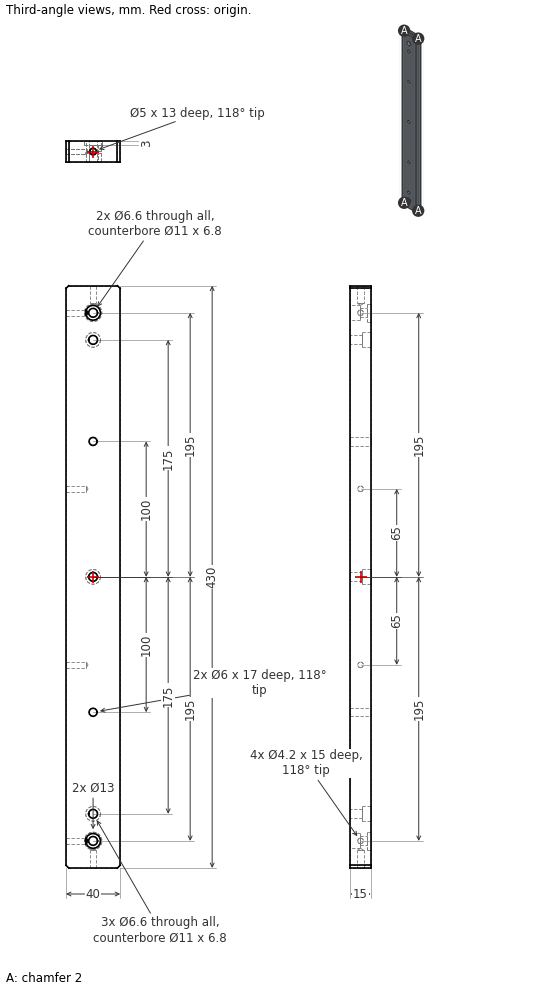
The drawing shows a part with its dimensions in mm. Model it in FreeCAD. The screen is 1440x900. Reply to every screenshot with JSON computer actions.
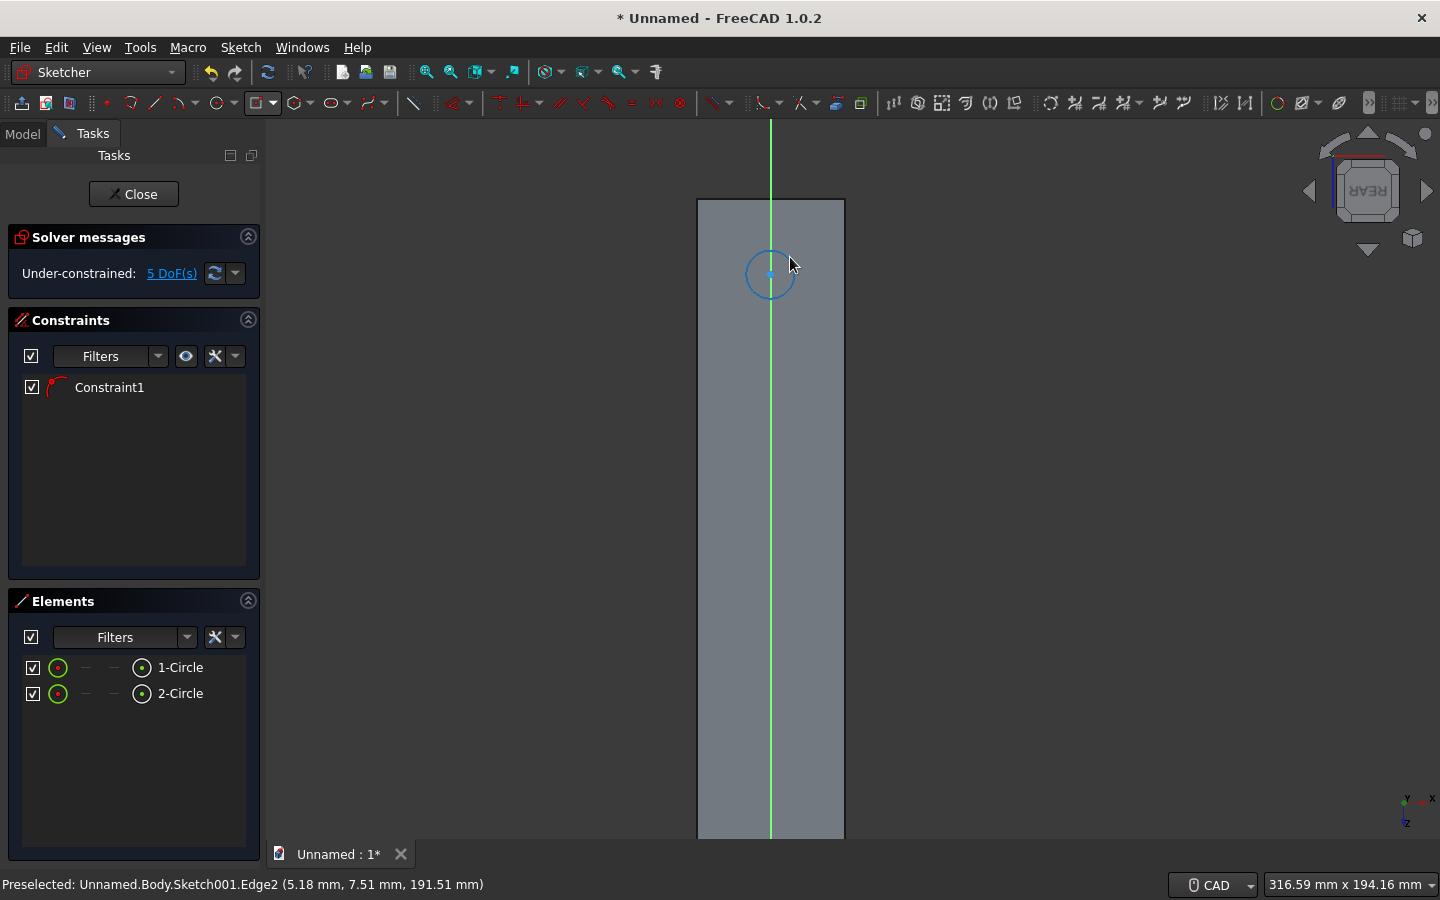
{"action": "left_click", "coordinate": [787, 258]}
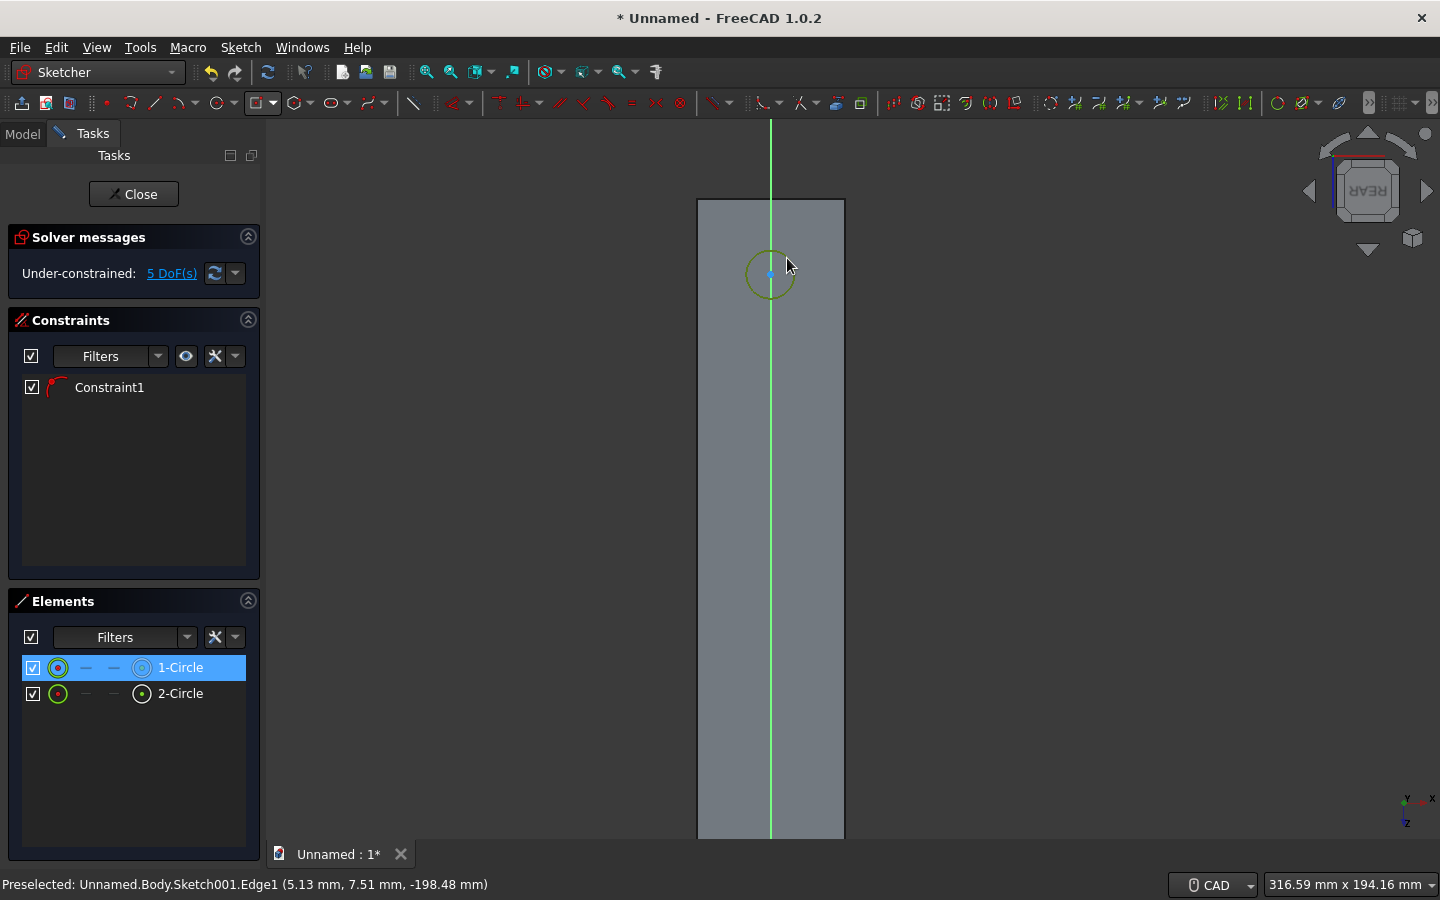
{"action": "scroll", "coordinate": [790, 256], "scroll_direction": "down", "scroll_amount": 6}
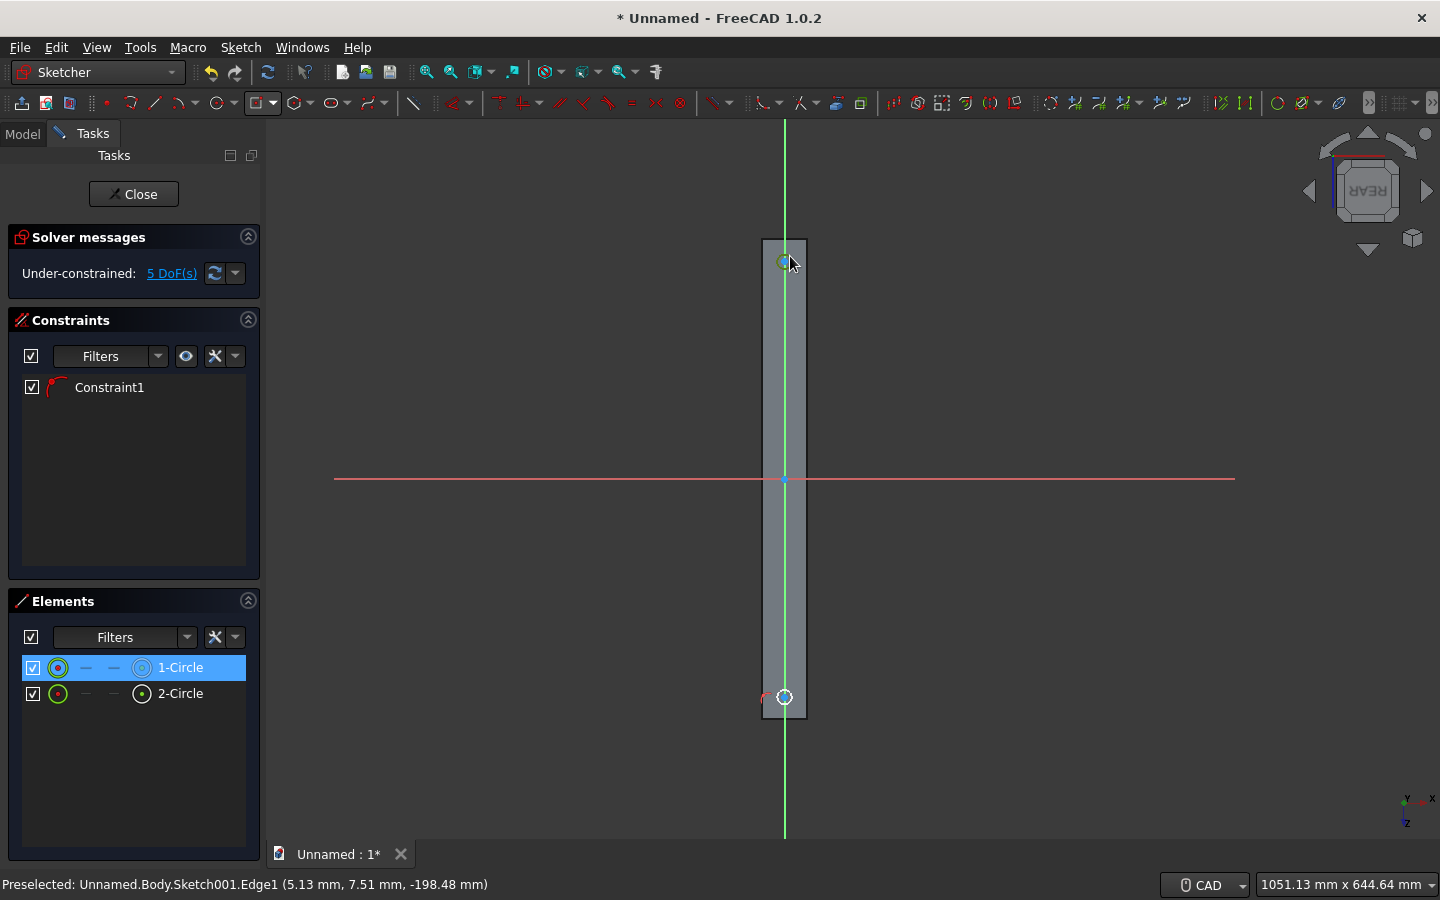
{"action": "scroll", "coordinate": [790, 692], "scroll_direction": "up", "scroll_amount": 6}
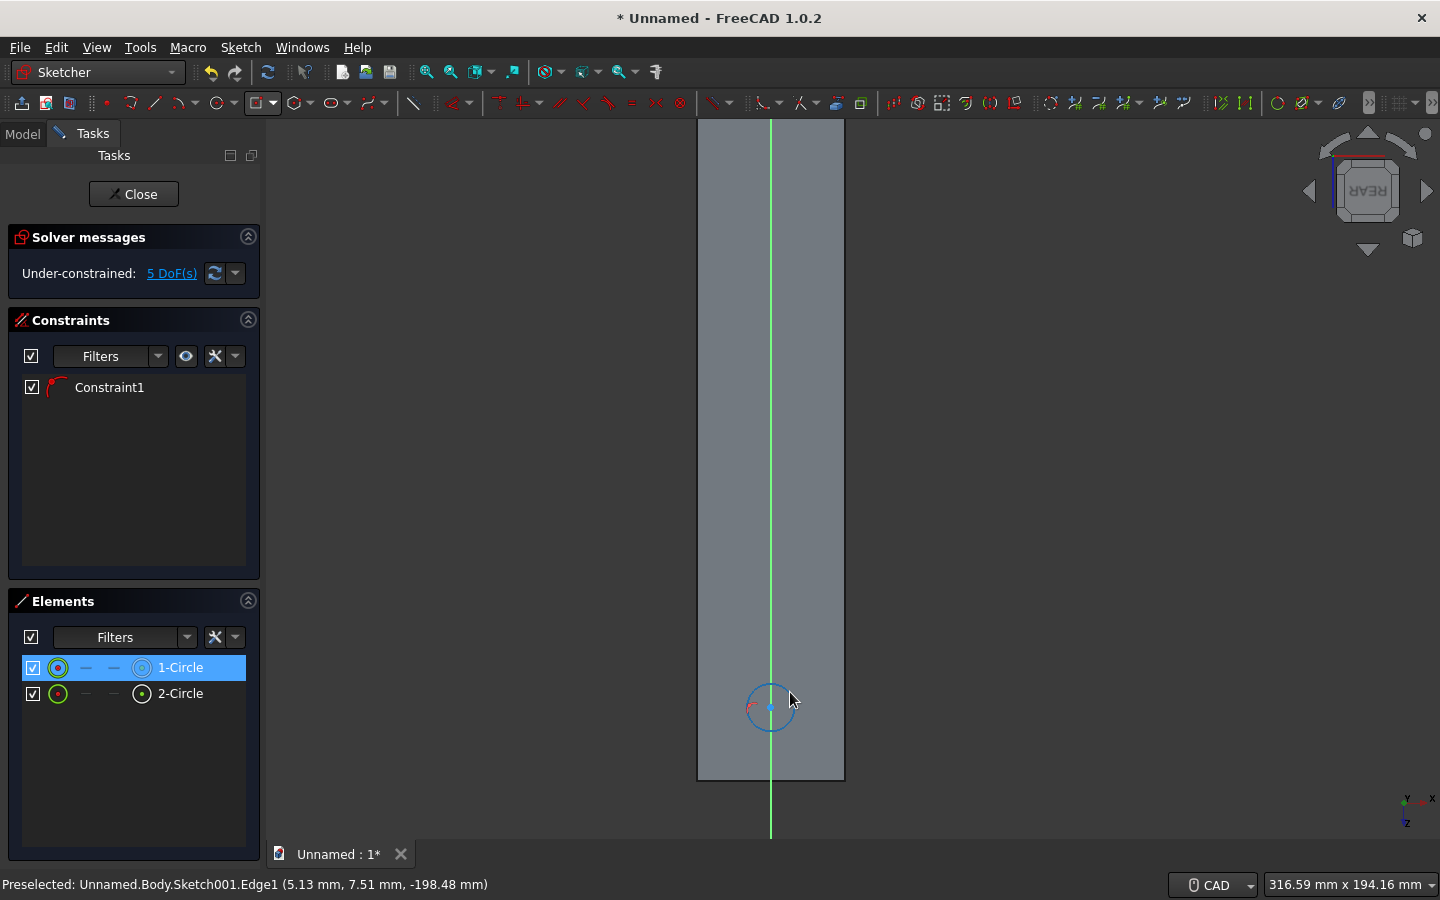
{"action": "left_click", "coordinate": [788, 691]}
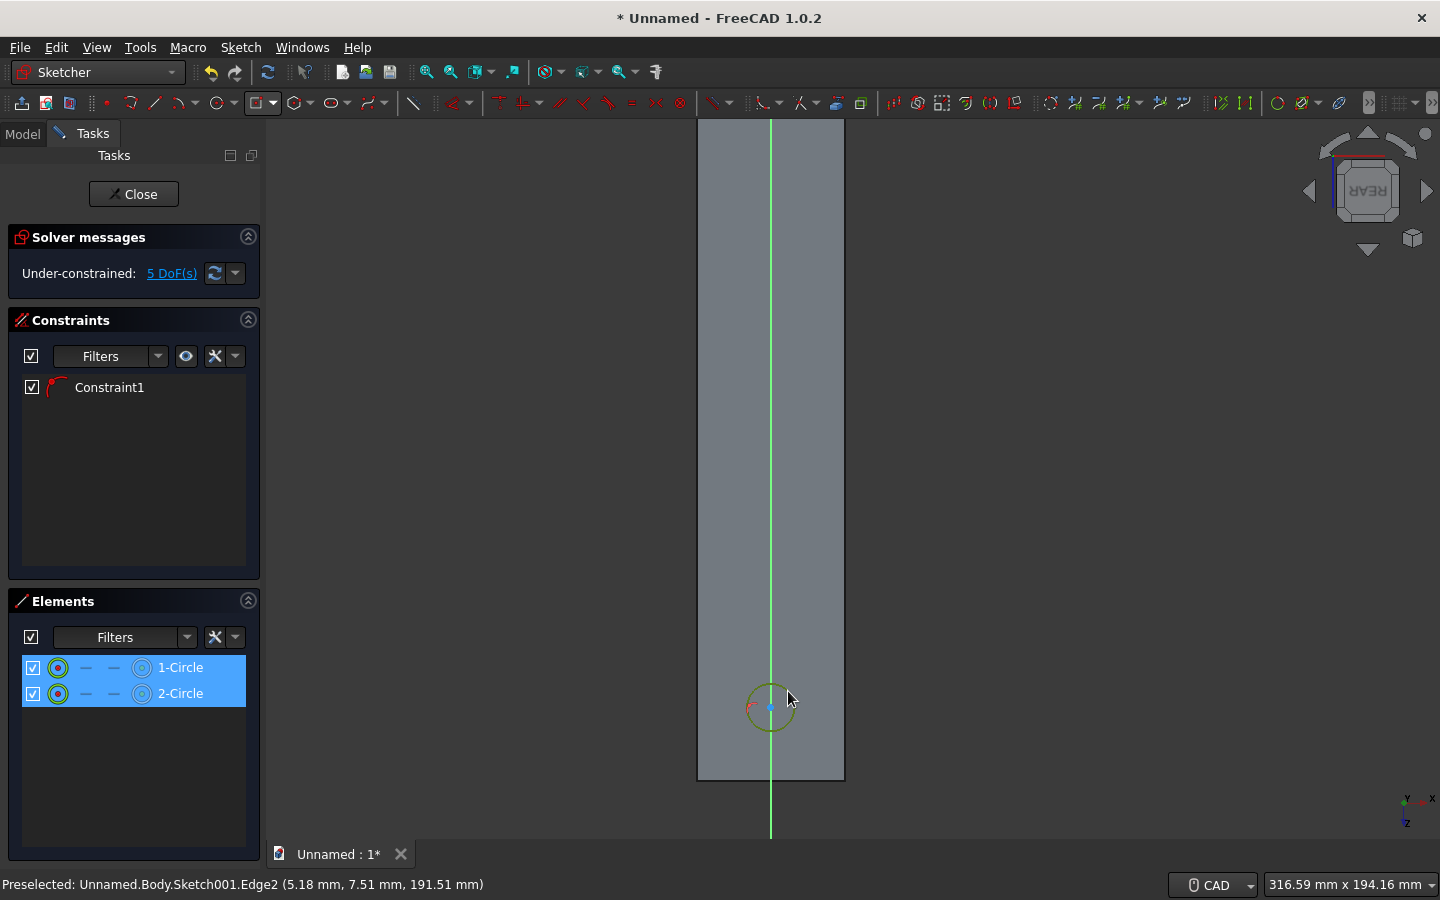
{"action": "key", "text": "e"}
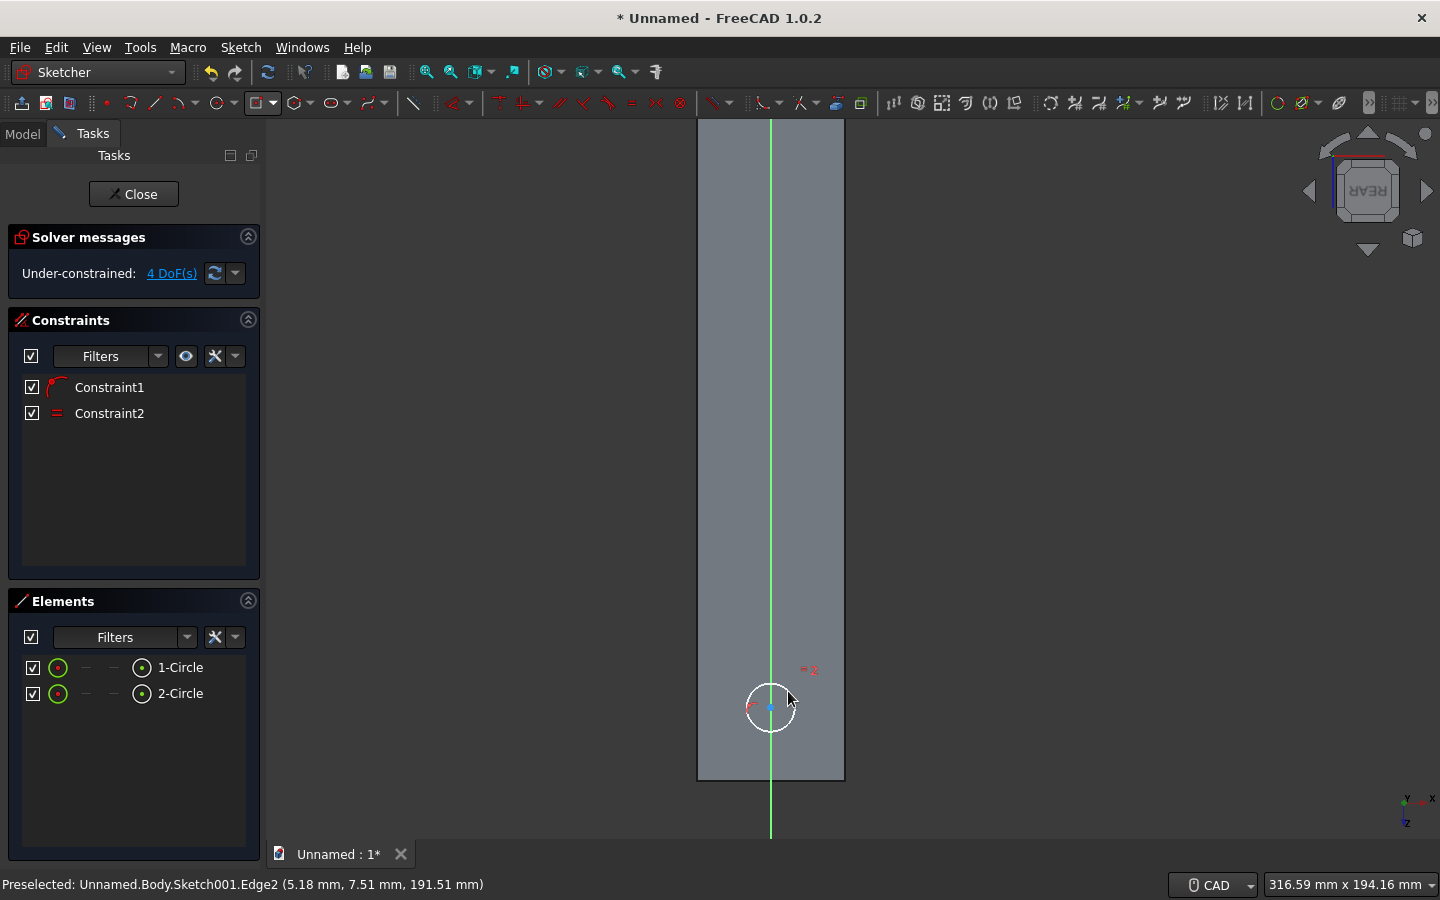
{"action": "scroll", "coordinate": [790, 693], "scroll_direction": "down", "scroll_amount": 6}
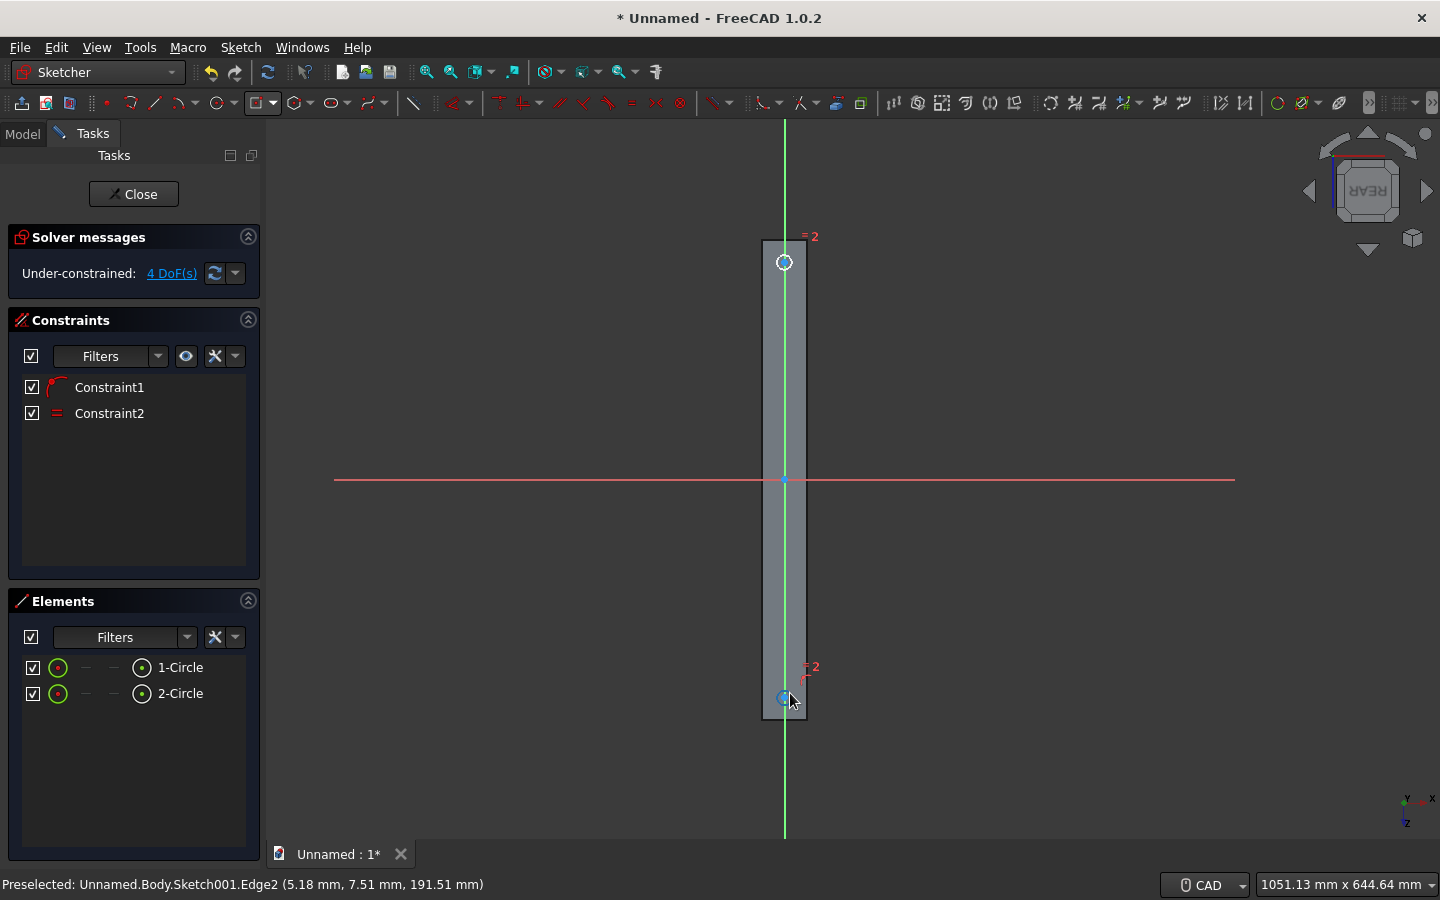
{"action": "left_click", "coordinate": [784, 262]}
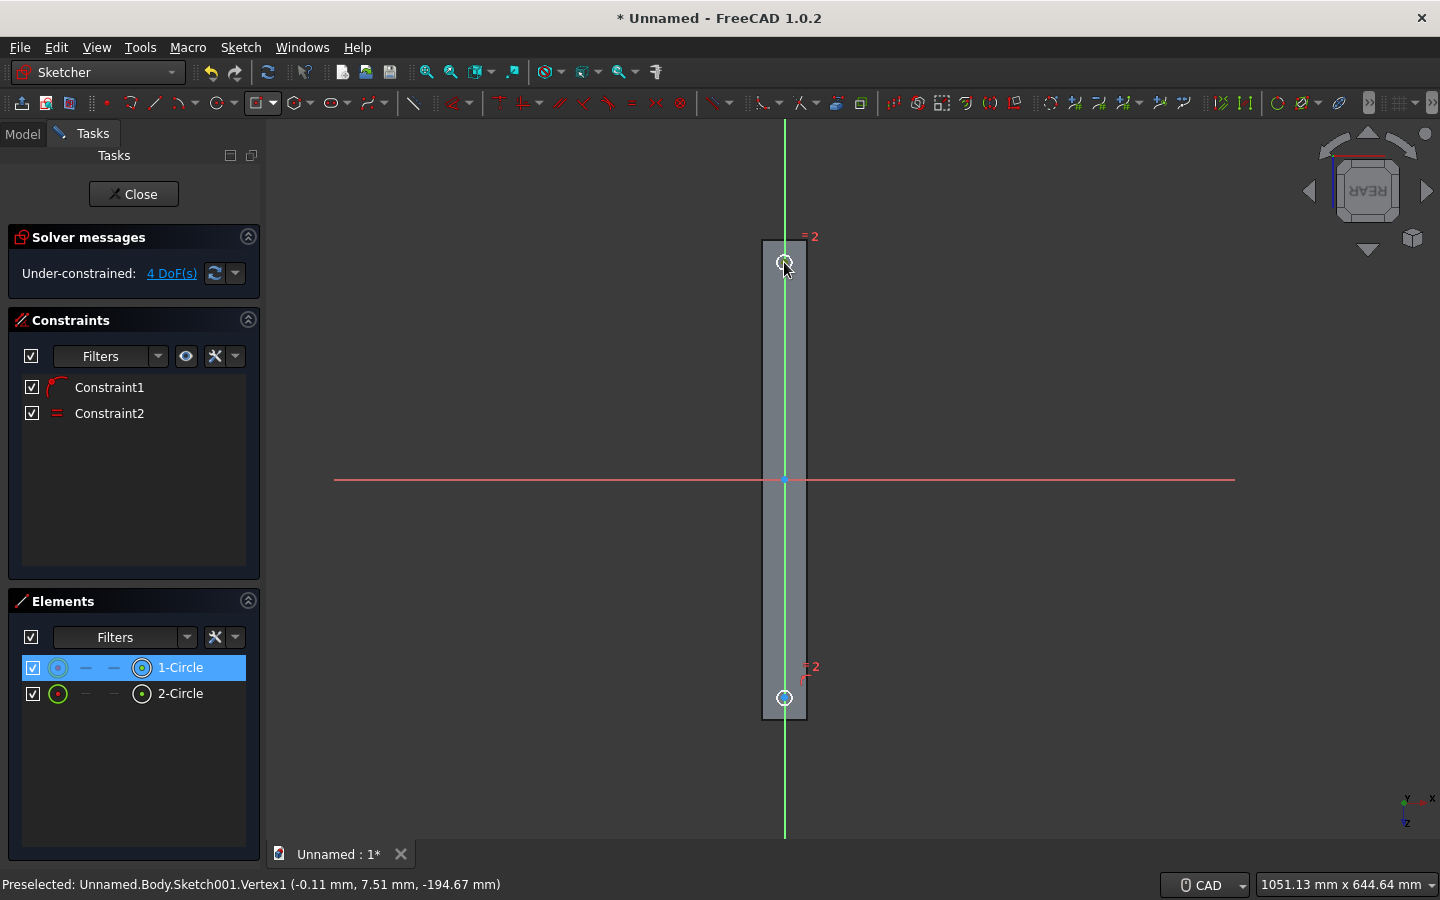
{"action": "left_click", "coordinate": [785, 764]}